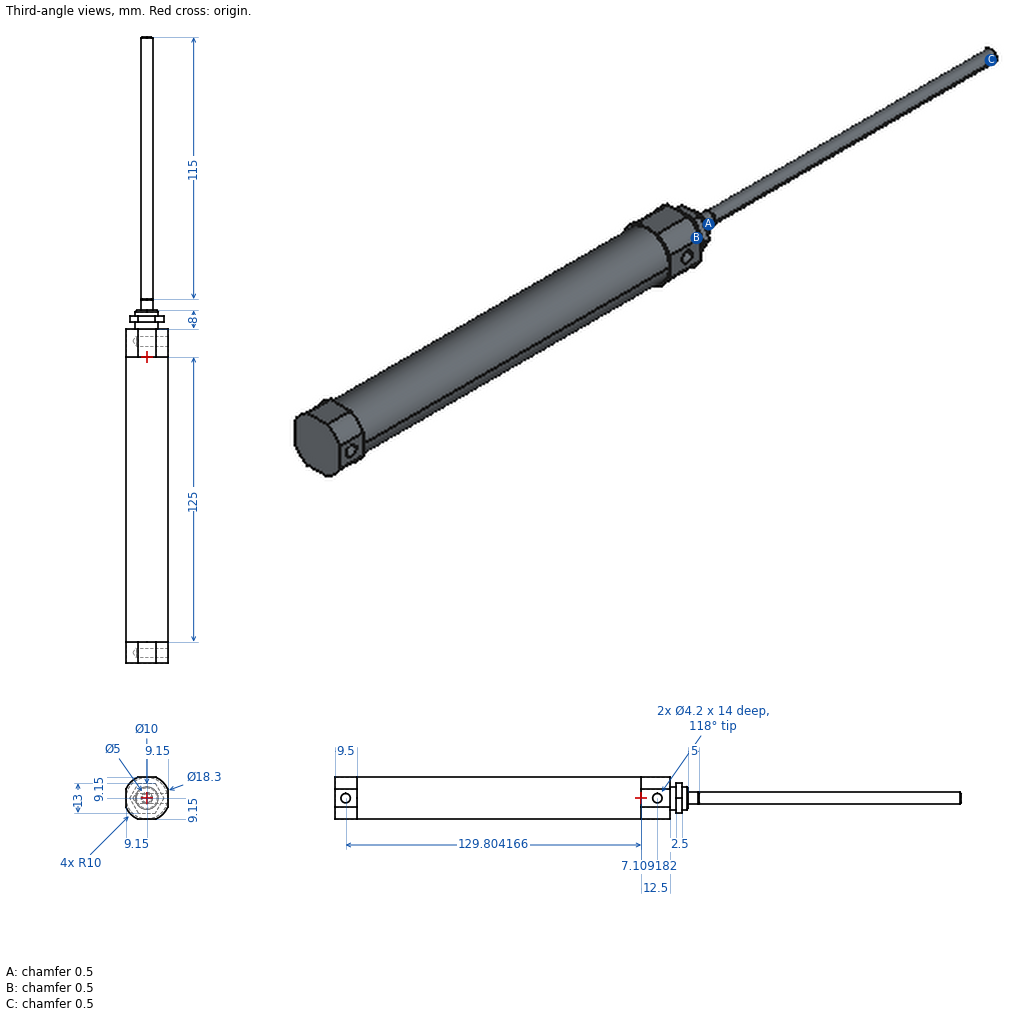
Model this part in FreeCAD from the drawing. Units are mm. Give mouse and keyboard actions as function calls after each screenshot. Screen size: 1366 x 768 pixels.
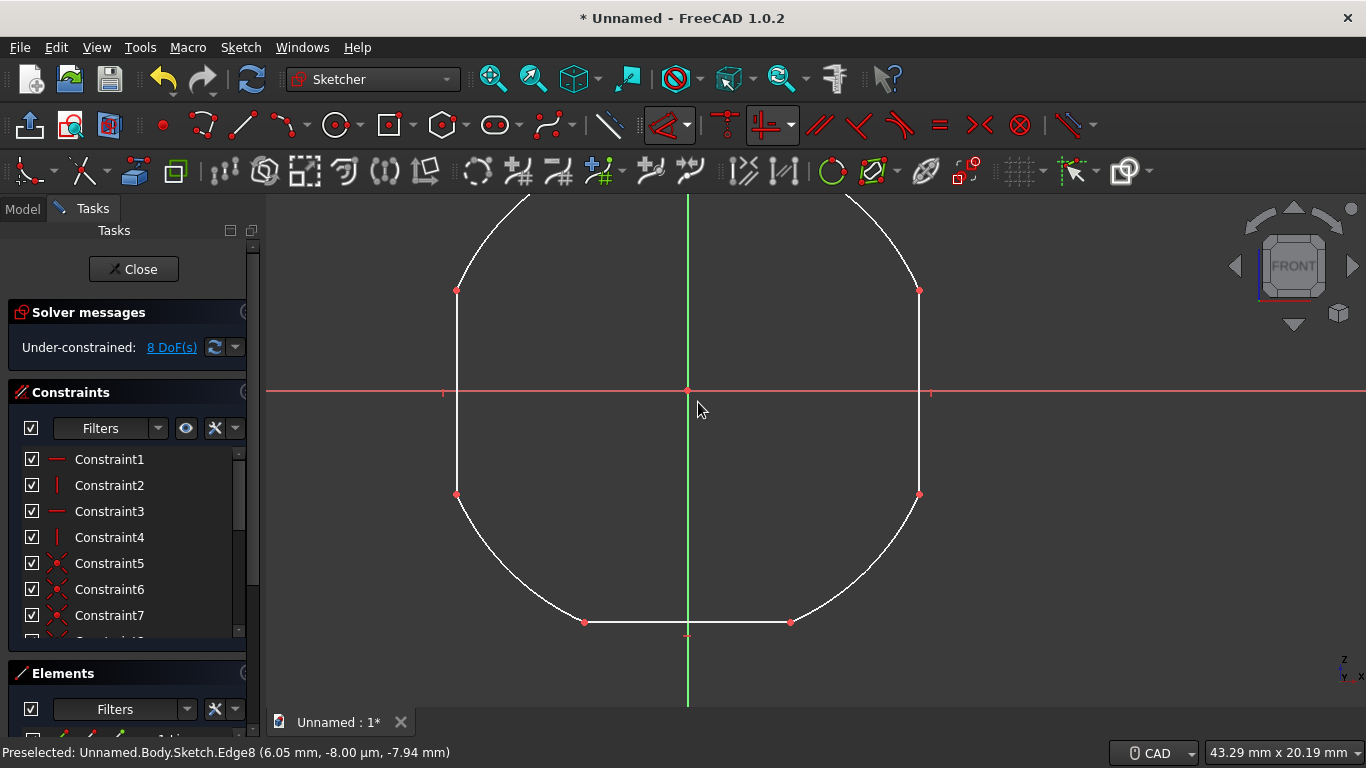
click(485, 542)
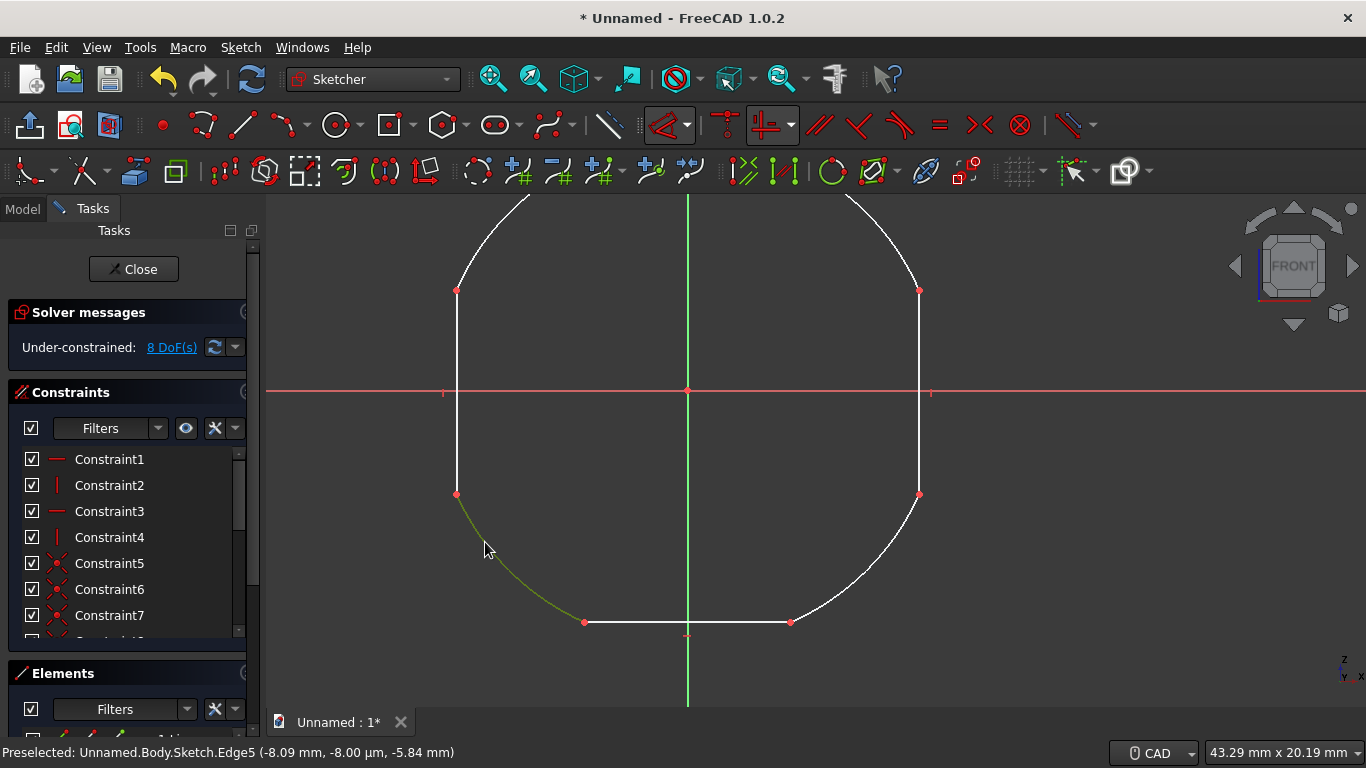
click(484, 242)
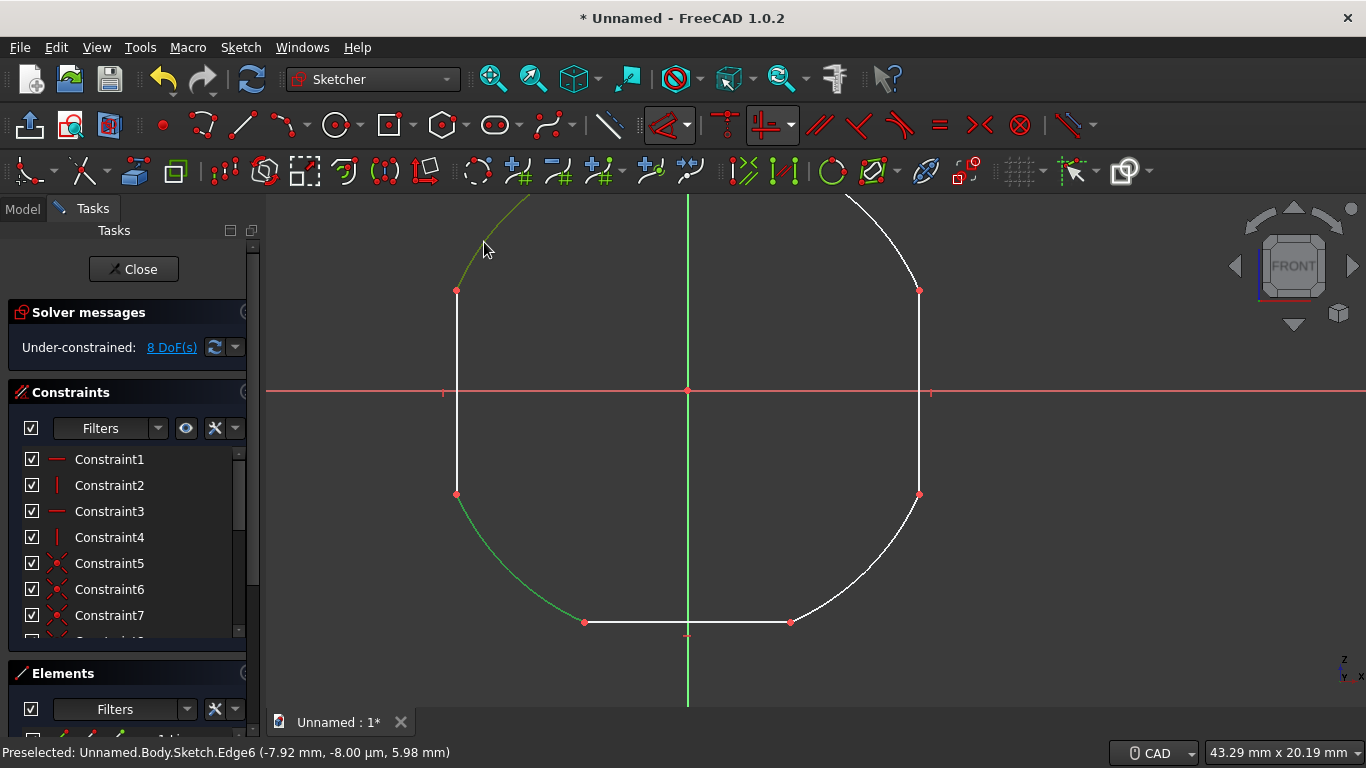
click(891, 242)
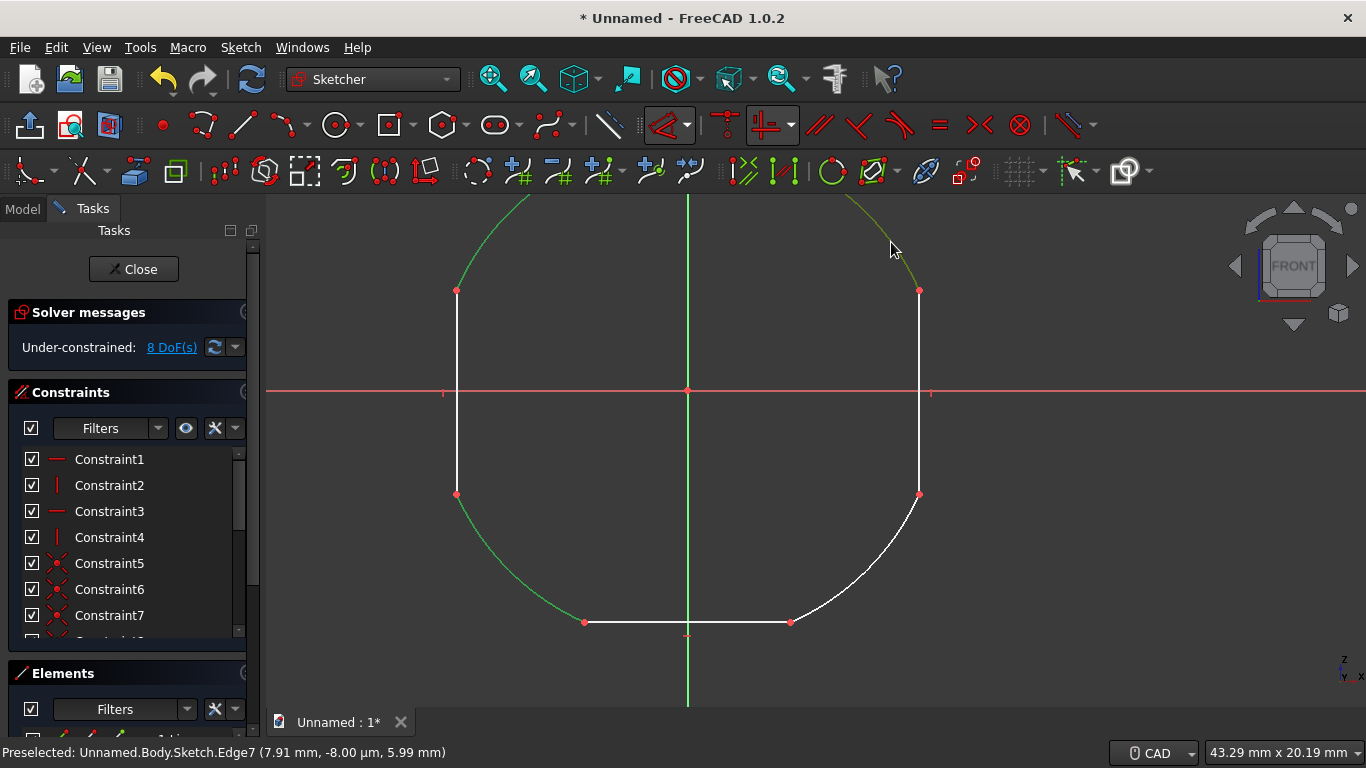
click(839, 595)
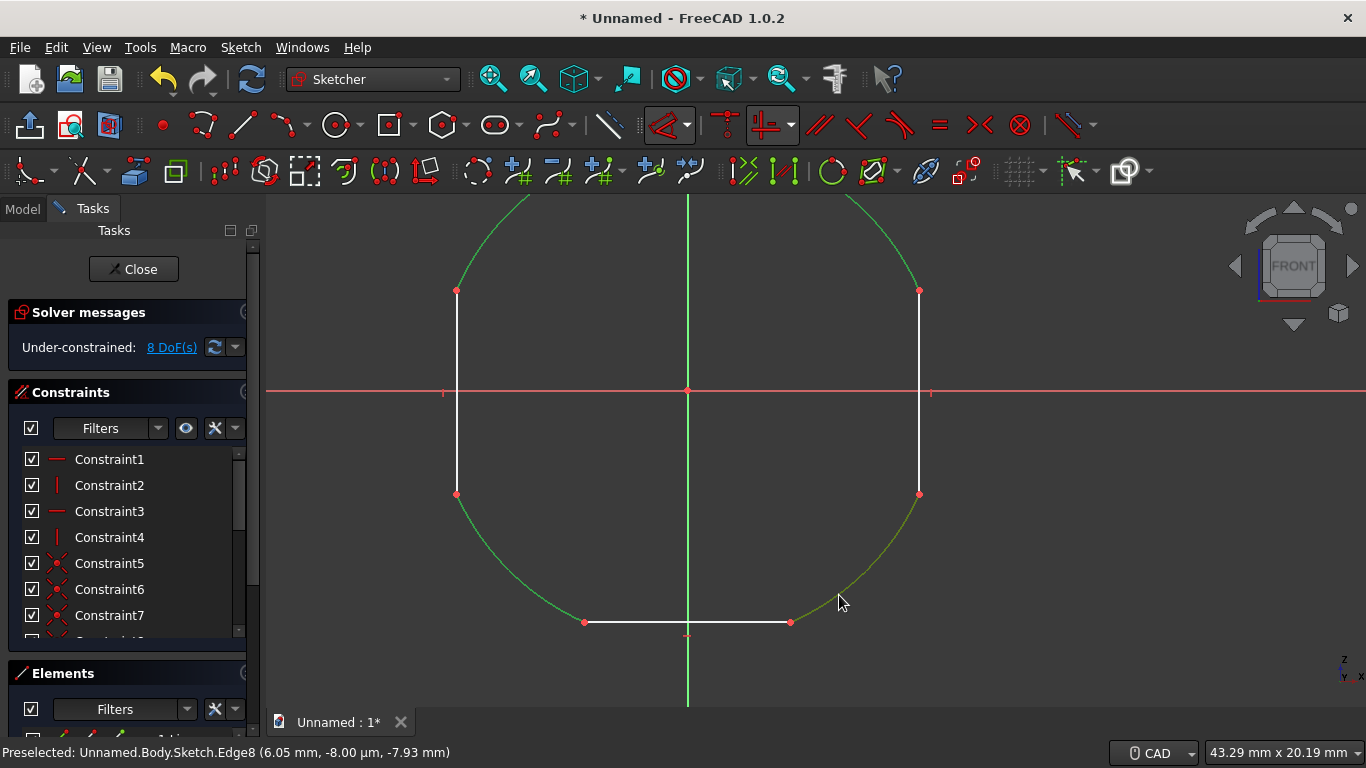
key(e)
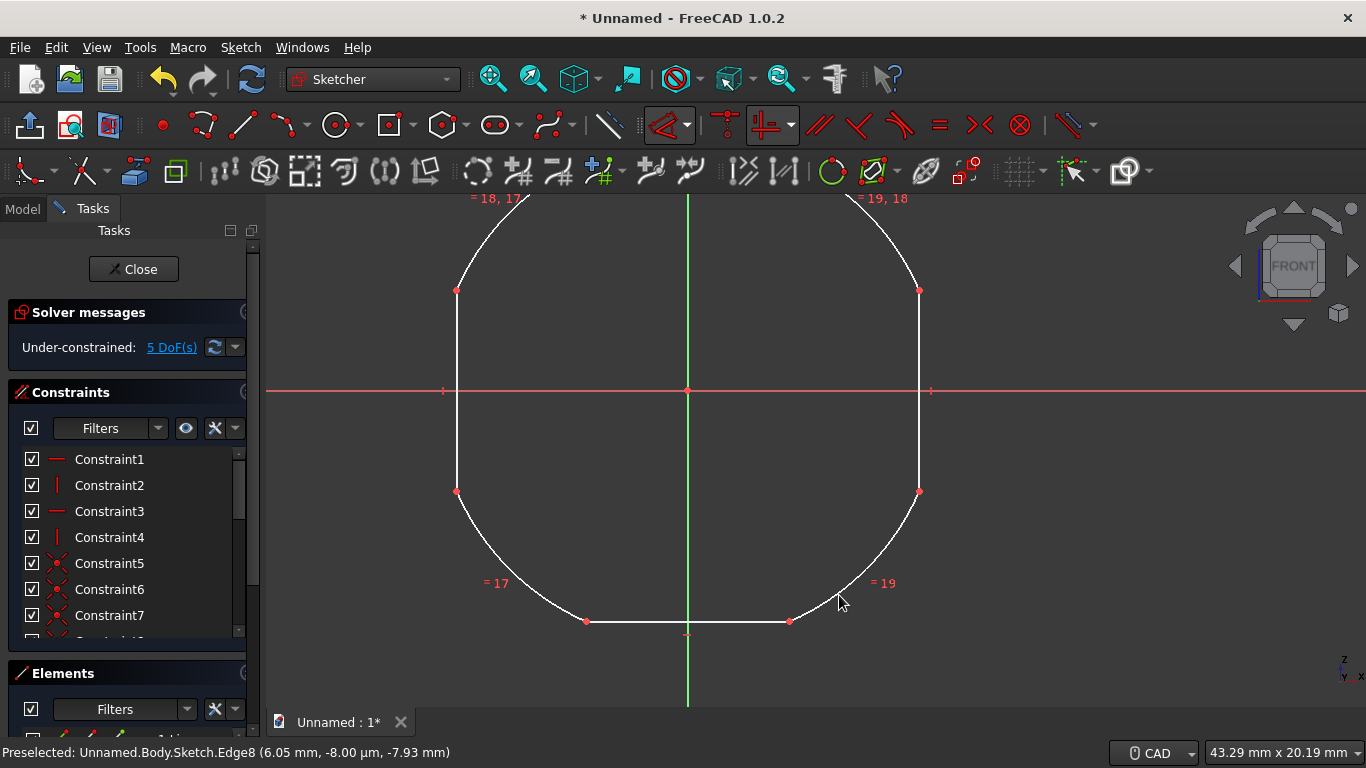
key(d)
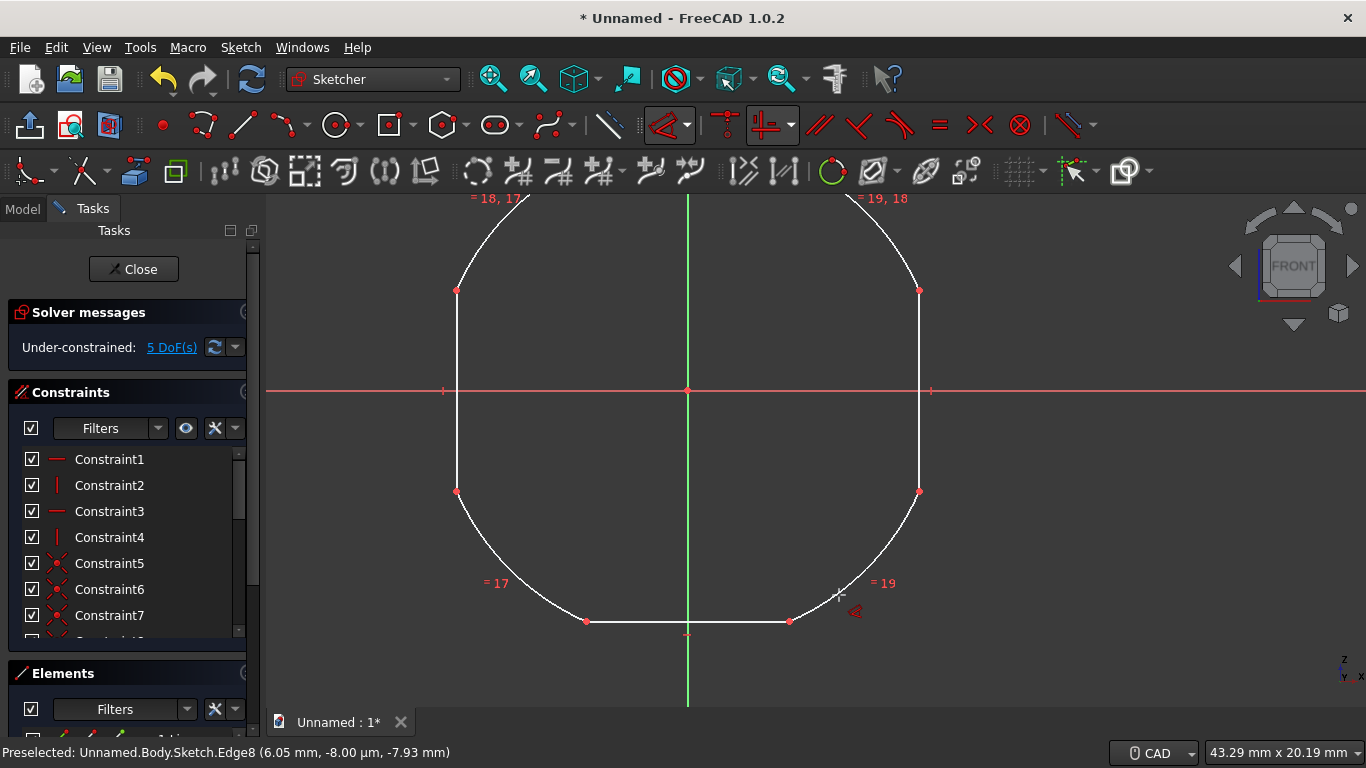
click(485, 540)
click(459, 559)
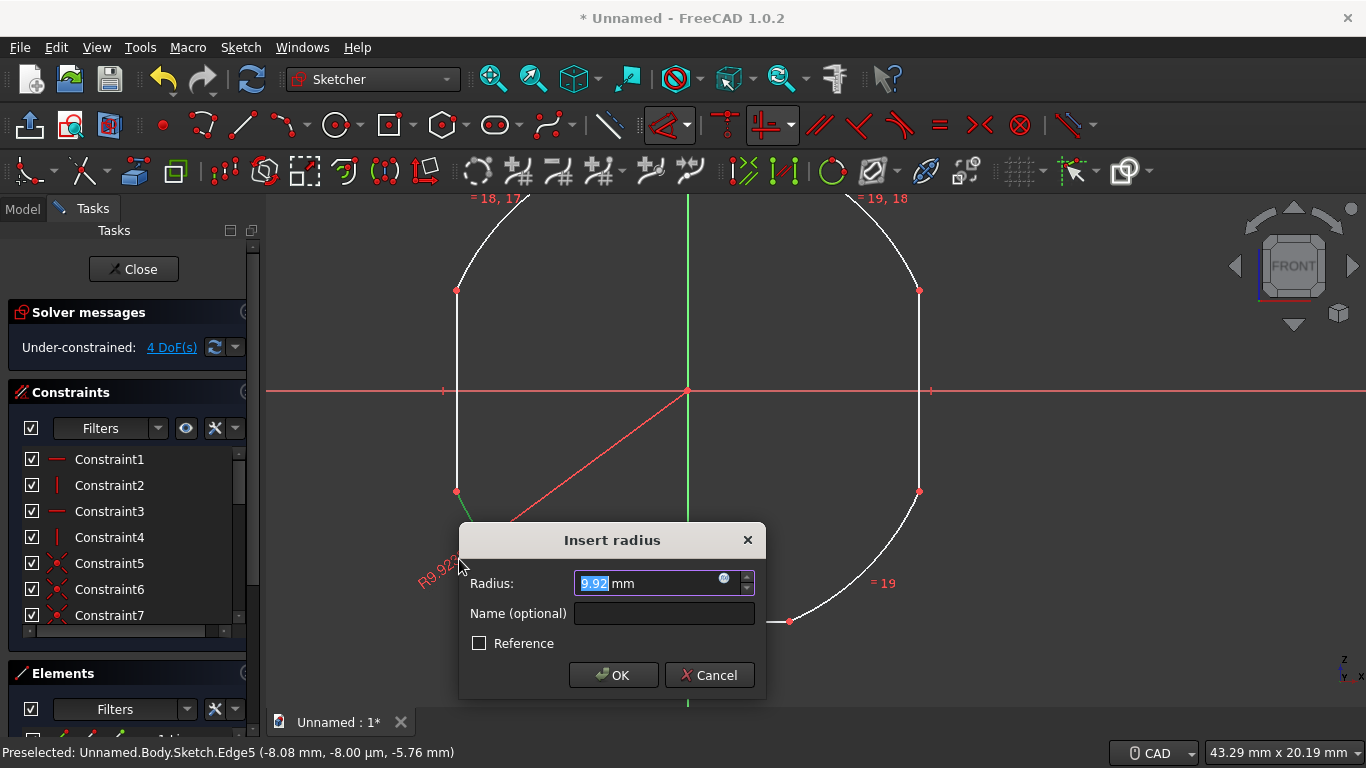
text(10)
key(Return)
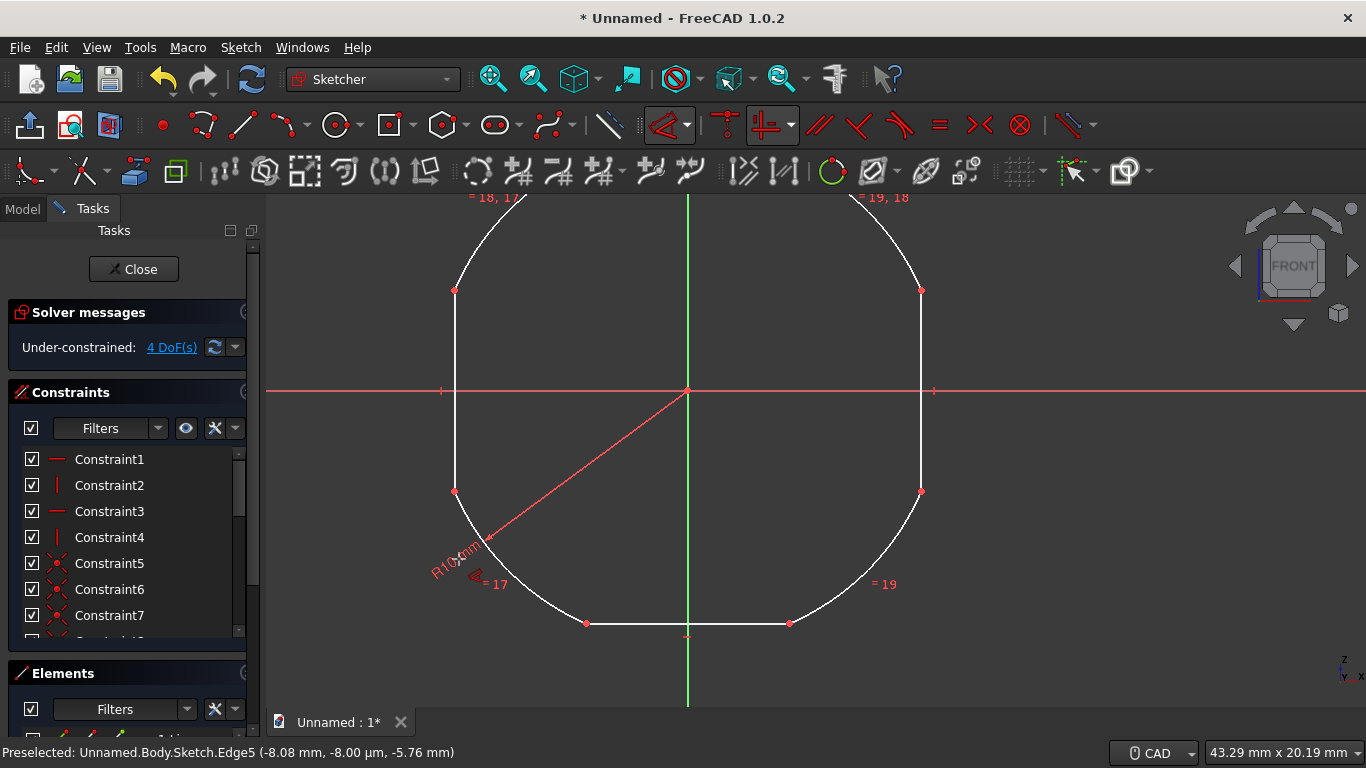
click(789, 624)
click(823, 507)